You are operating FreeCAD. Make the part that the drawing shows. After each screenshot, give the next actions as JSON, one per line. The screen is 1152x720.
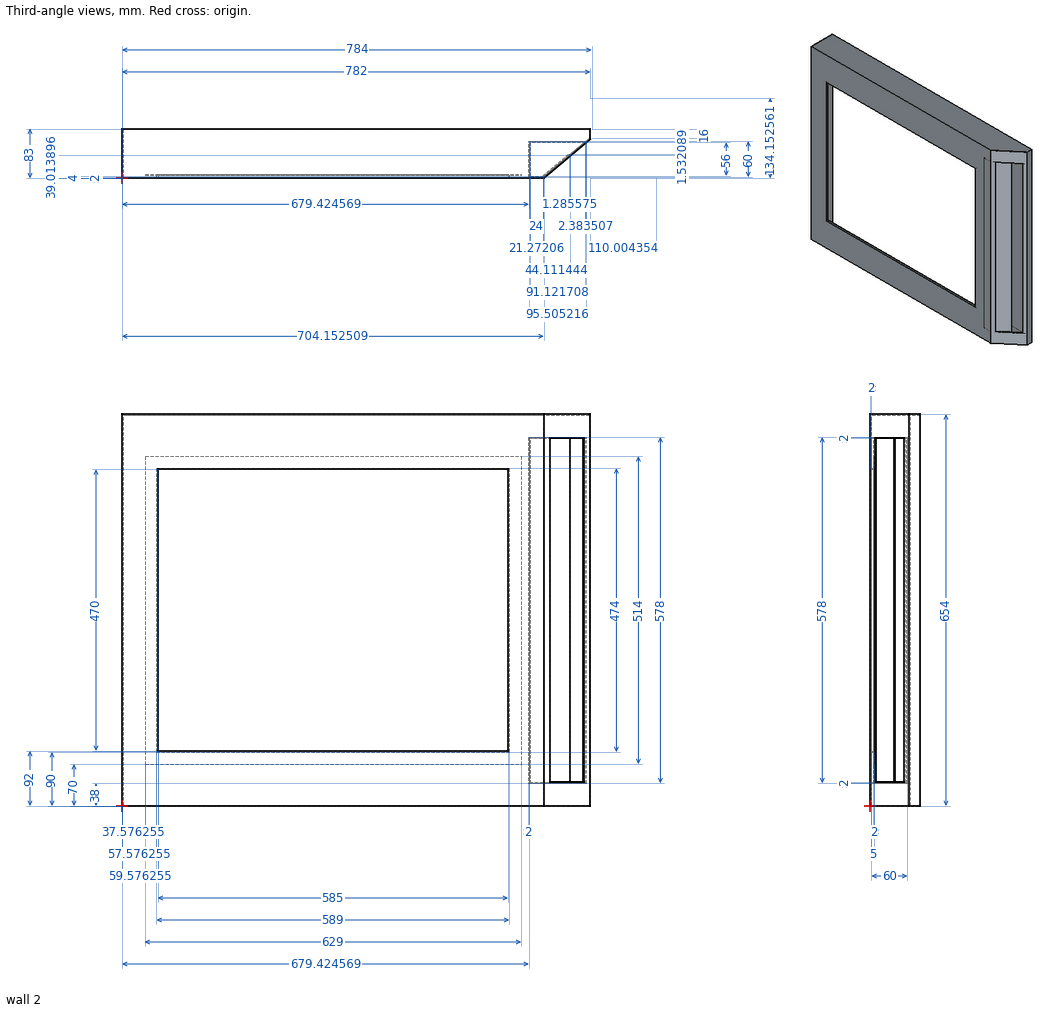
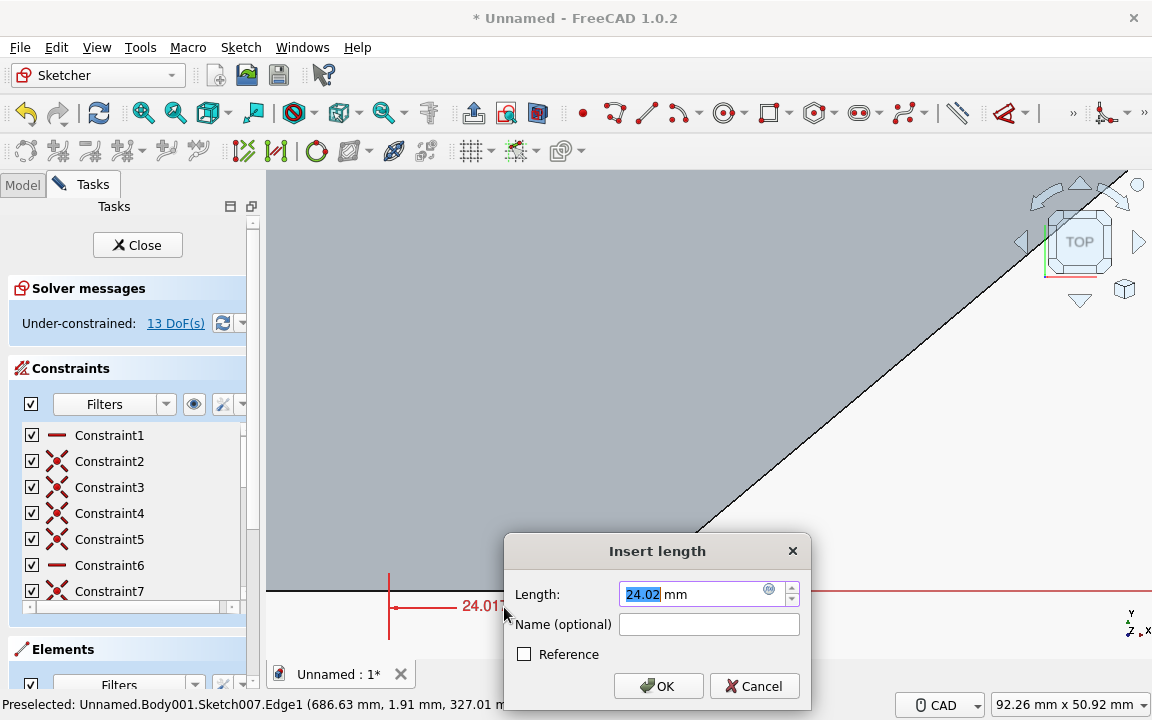
{"action": "type", "text": "24"}
{"action": "key", "text": "Return"}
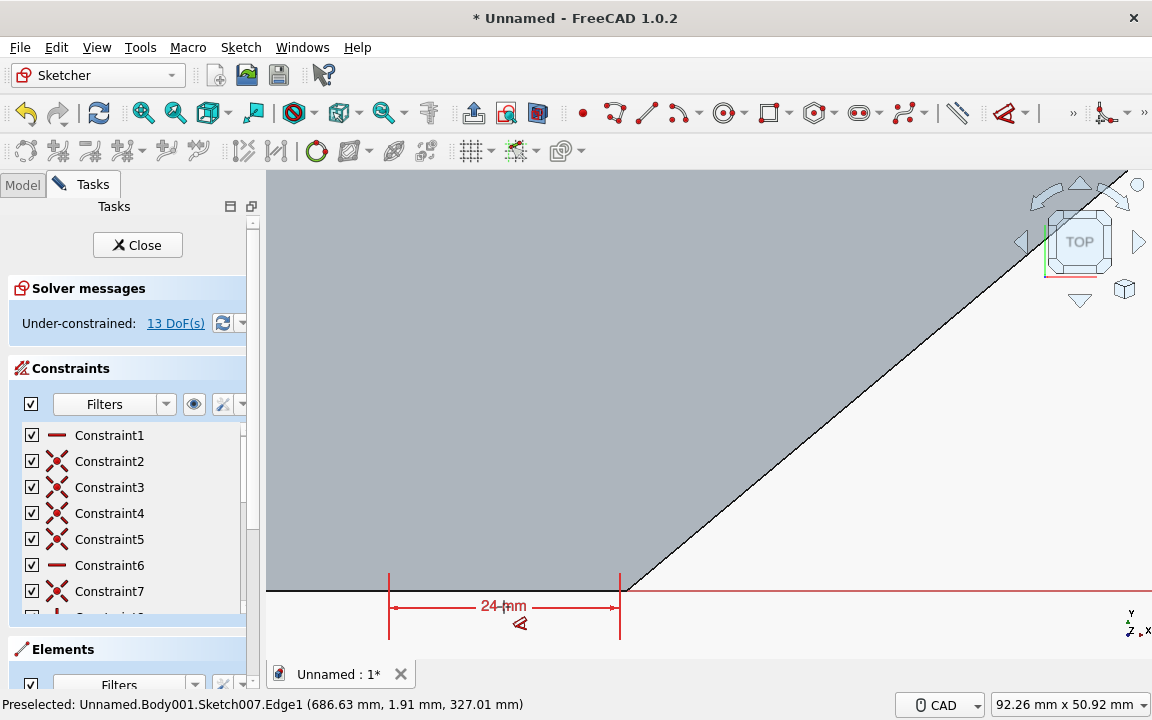
{"action": "left_click", "coordinate": [408, 393]}
{"action": "left_click", "coordinate": [374, 376]}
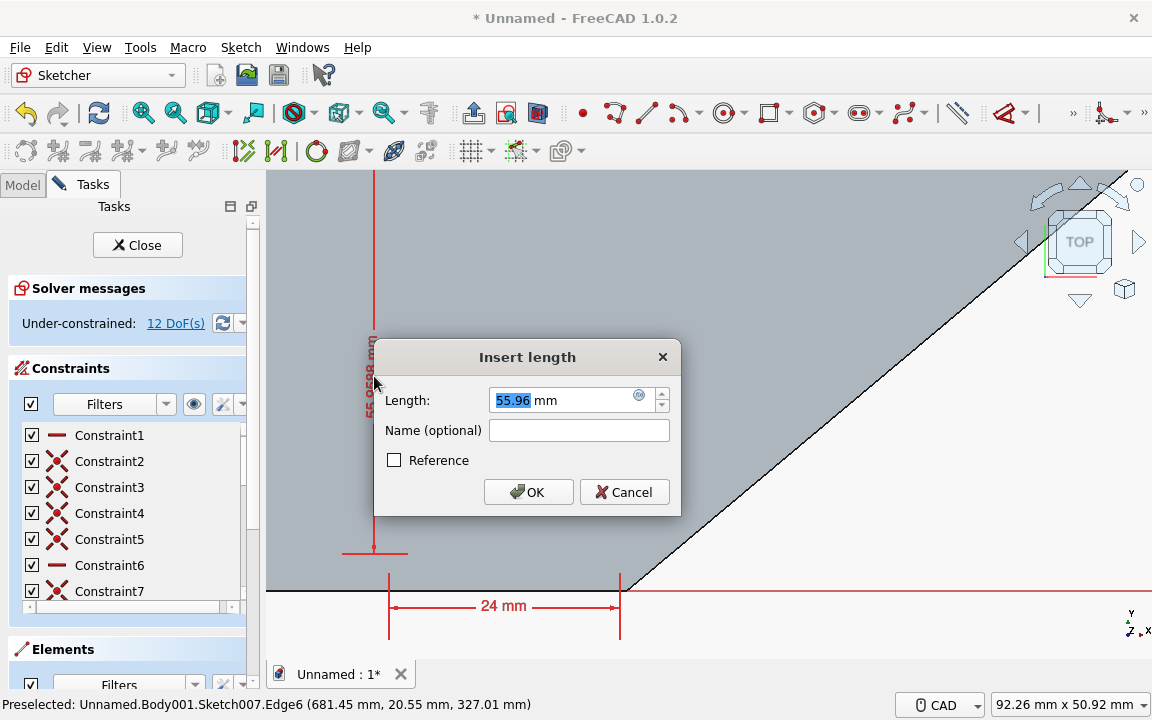
{"action": "type", "text": "56"}
{"action": "key", "text": "Return"}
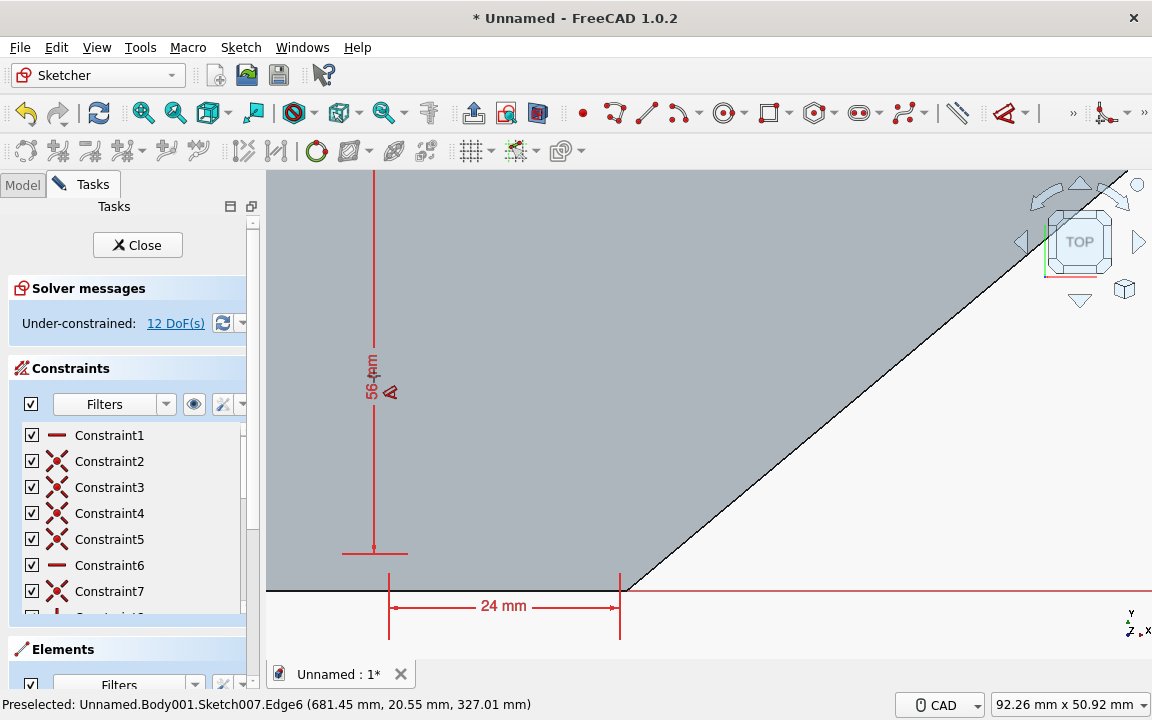
{"action": "left_click", "coordinate": [389, 401]}
{"action": "left_click", "coordinate": [355, 299]}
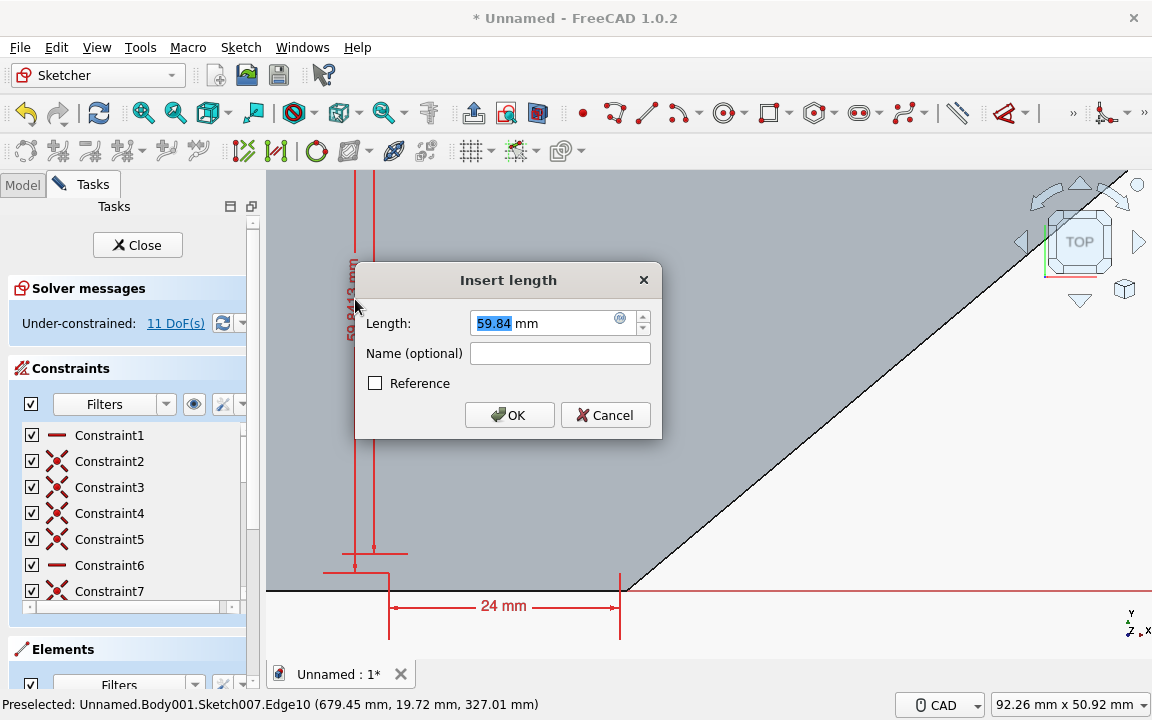
{"action": "type", "text": "60"}
{"action": "key", "text": "Return"}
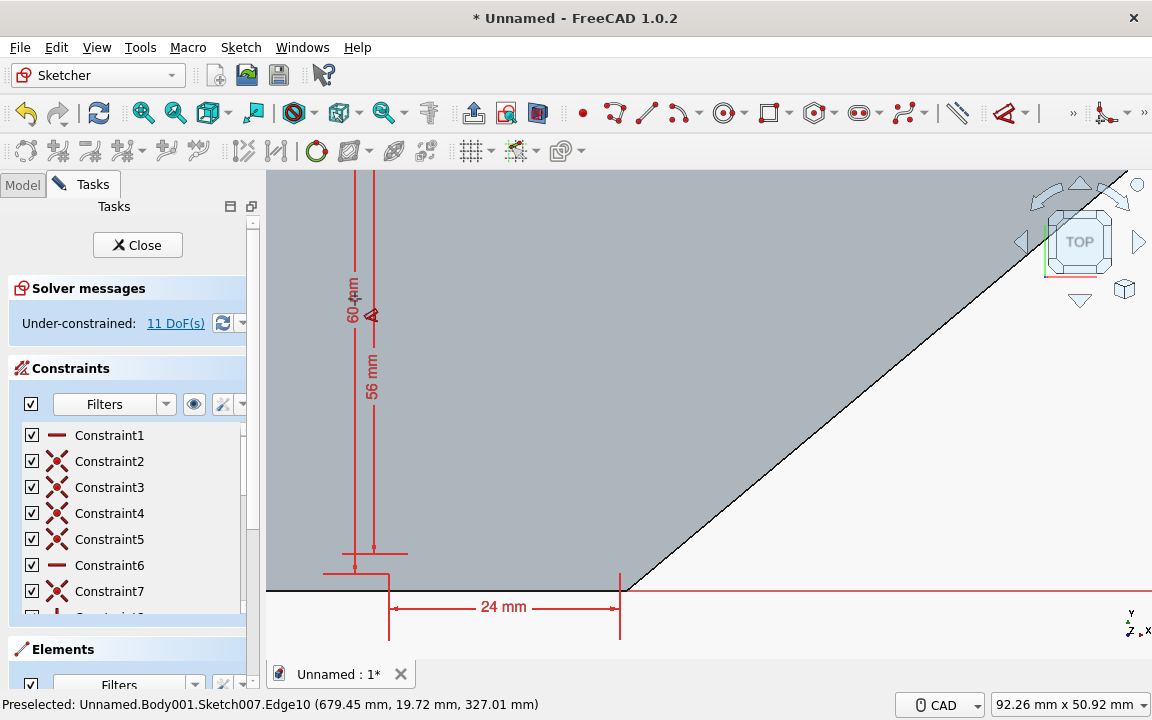
{"action": "scroll", "coordinate": [389, 574], "scroll_direction": "up", "scroll_amount": 4}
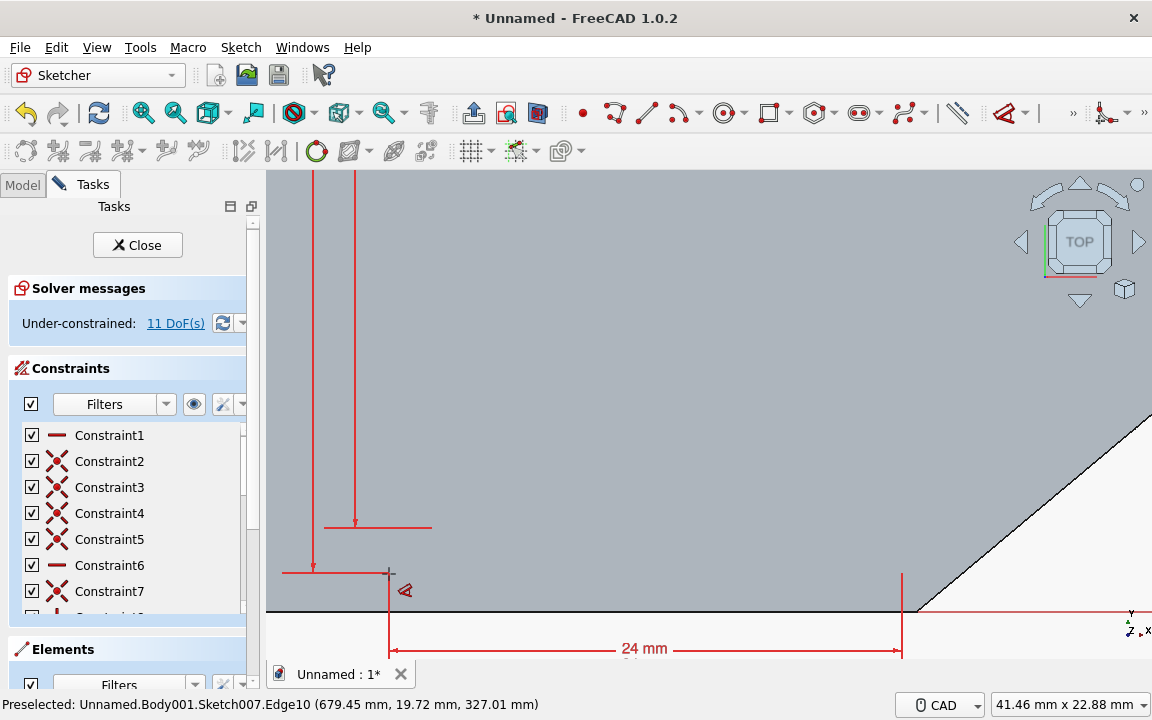
{"action": "left_click", "coordinate": [389, 573]}
{"action": "left_click", "coordinate": [423, 592]}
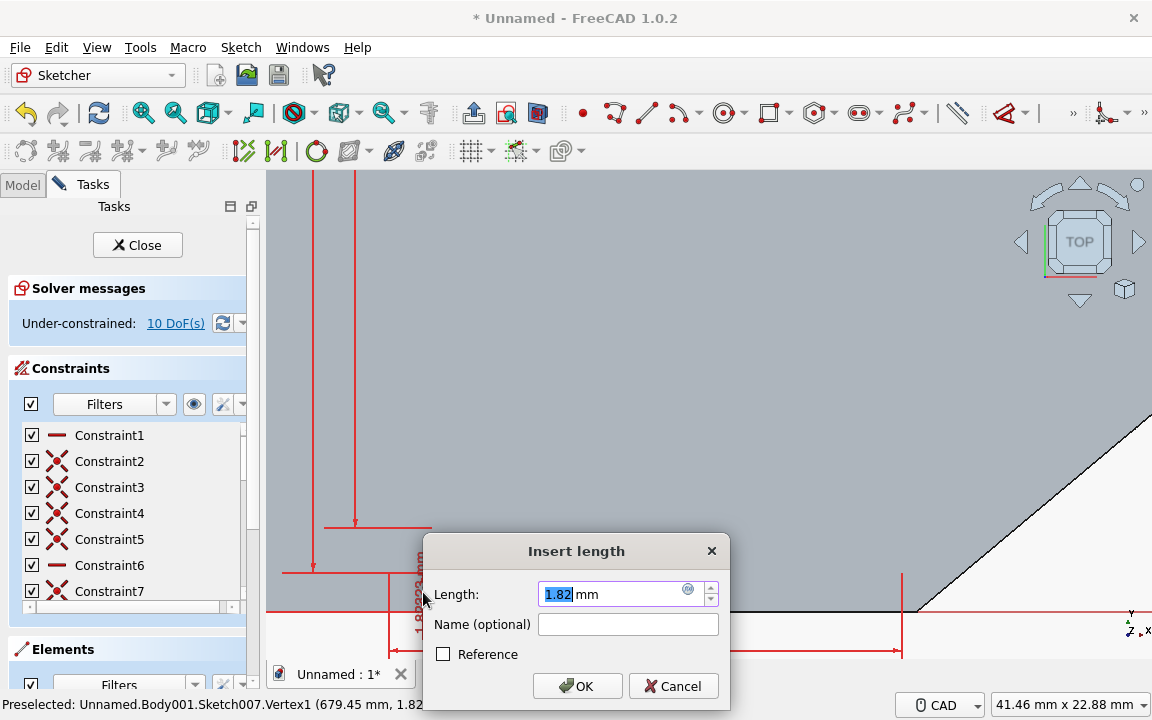
{"action": "type", "text": "2"}
{"action": "key", "text": "Return"}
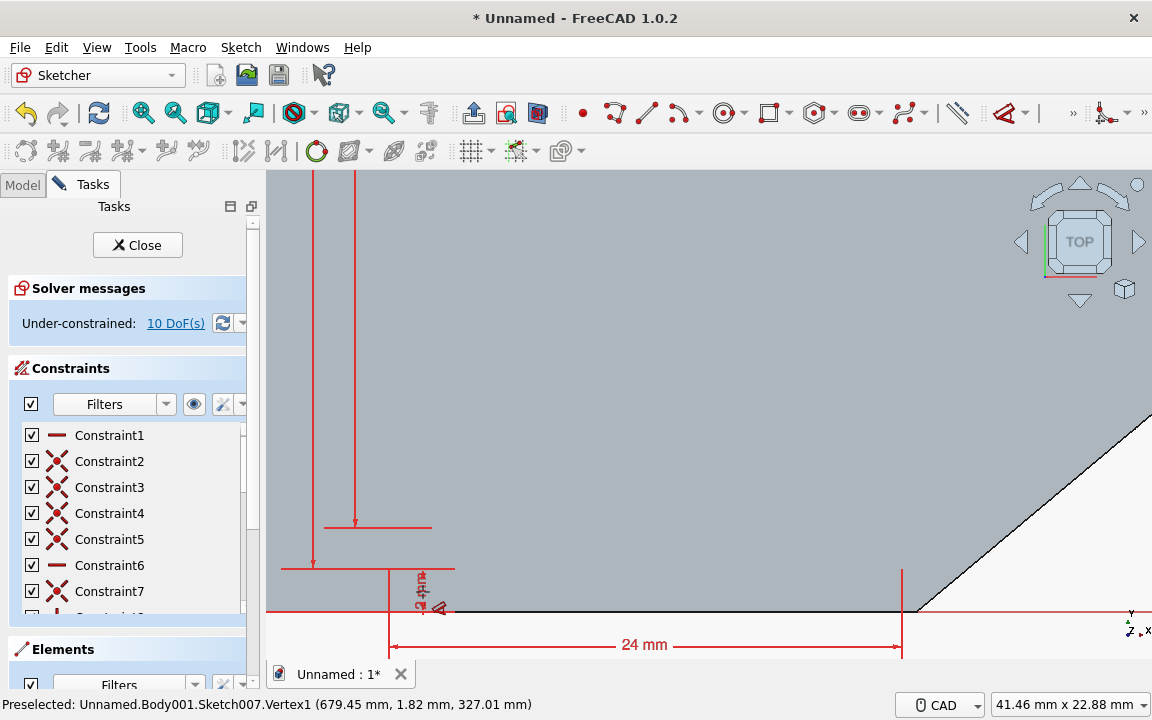
{"action": "left_click", "coordinate": [886, 528]}
{"action": "left_click", "coordinate": [920, 589]}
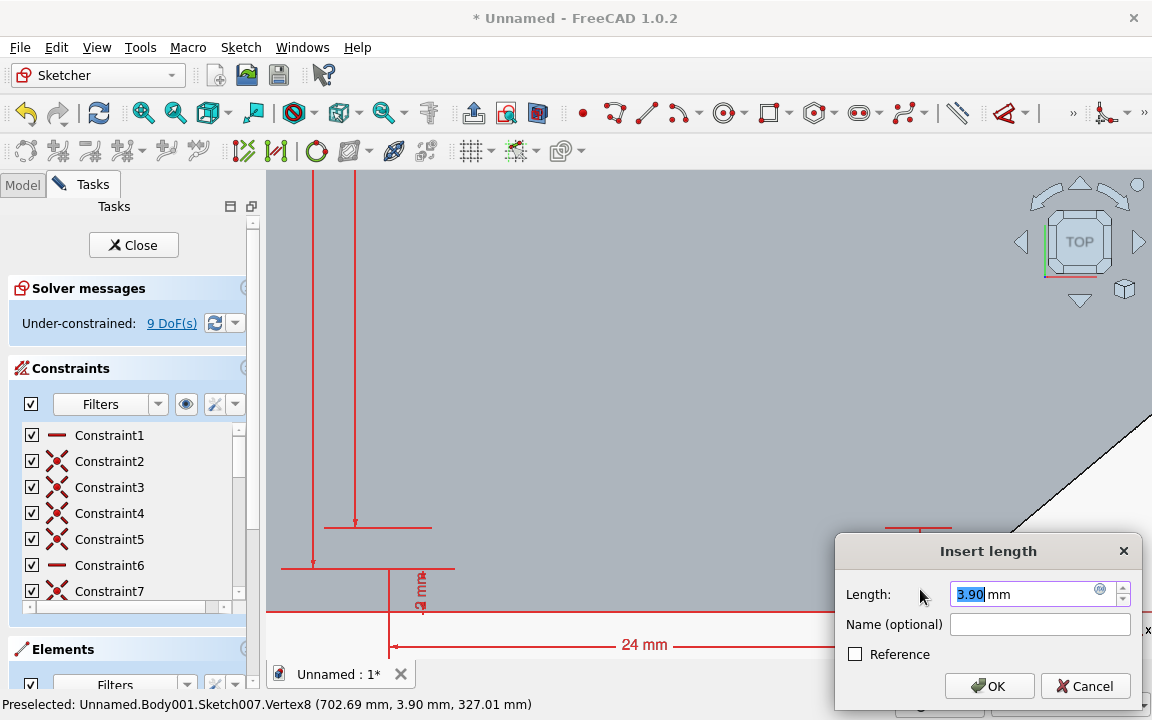
{"action": "type", "text": "4"}
{"action": "key", "text": "Return"}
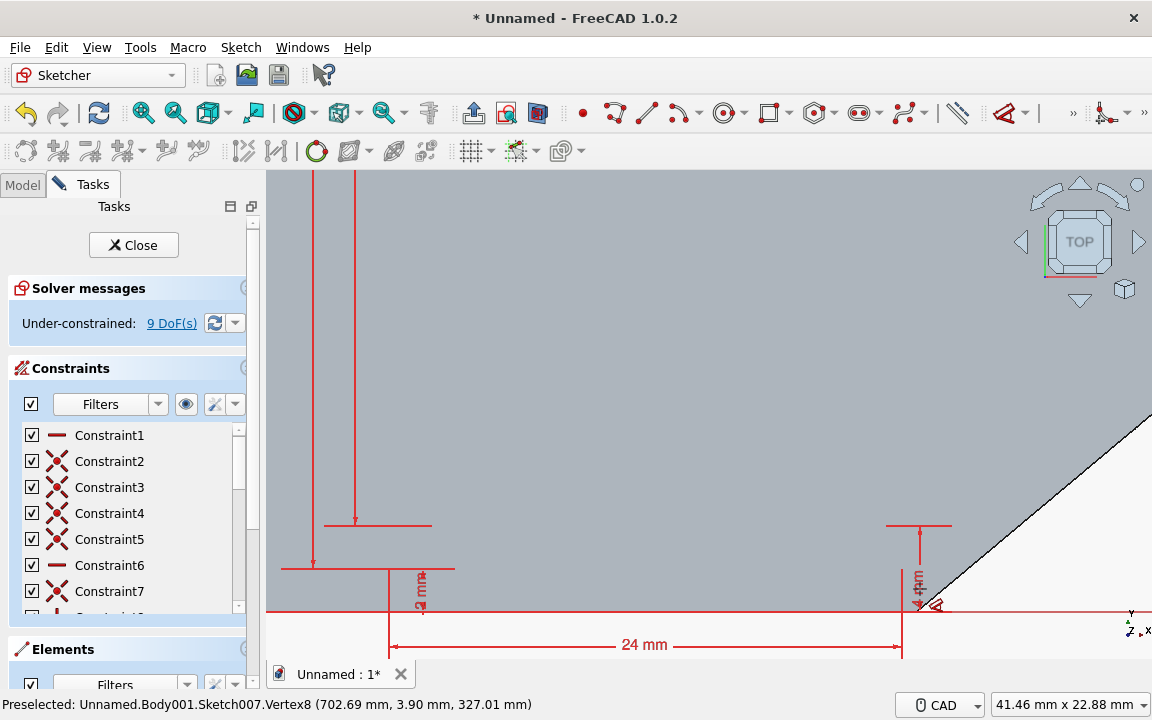
{"action": "scroll", "coordinate": [389, 574], "scroll_direction": "down", "scroll_amount": 7}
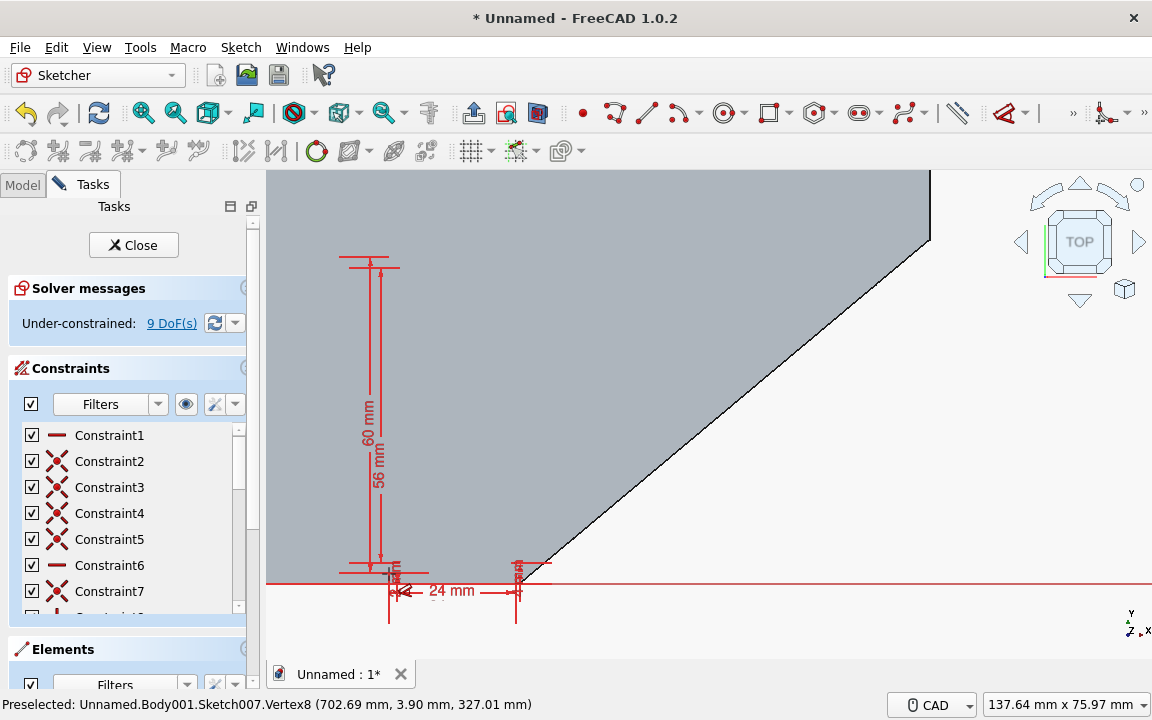
{"action": "scroll", "coordinate": [478, 563], "scroll_direction": "up", "scroll_amount": 2}